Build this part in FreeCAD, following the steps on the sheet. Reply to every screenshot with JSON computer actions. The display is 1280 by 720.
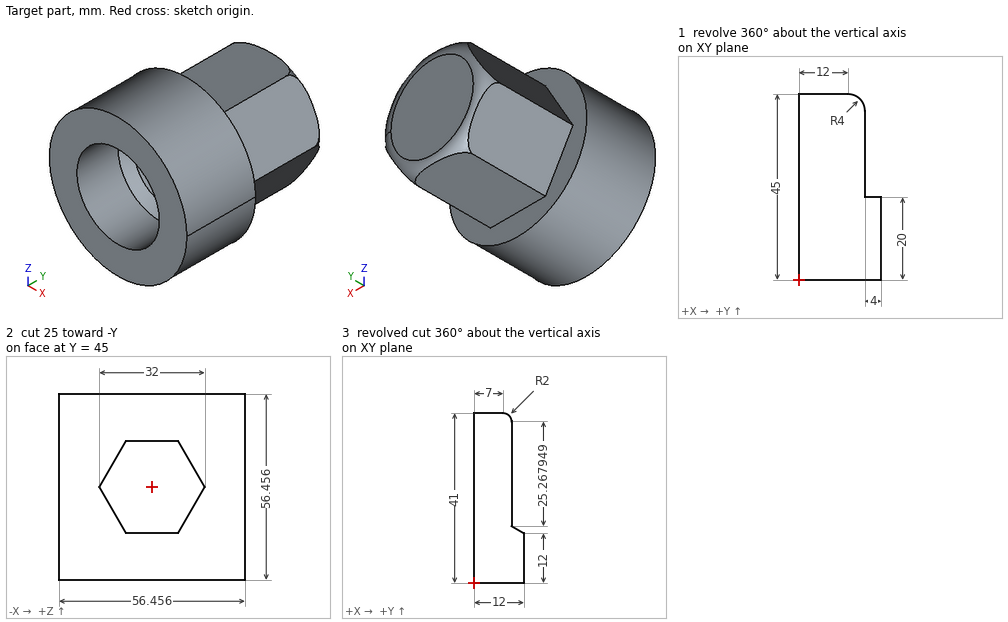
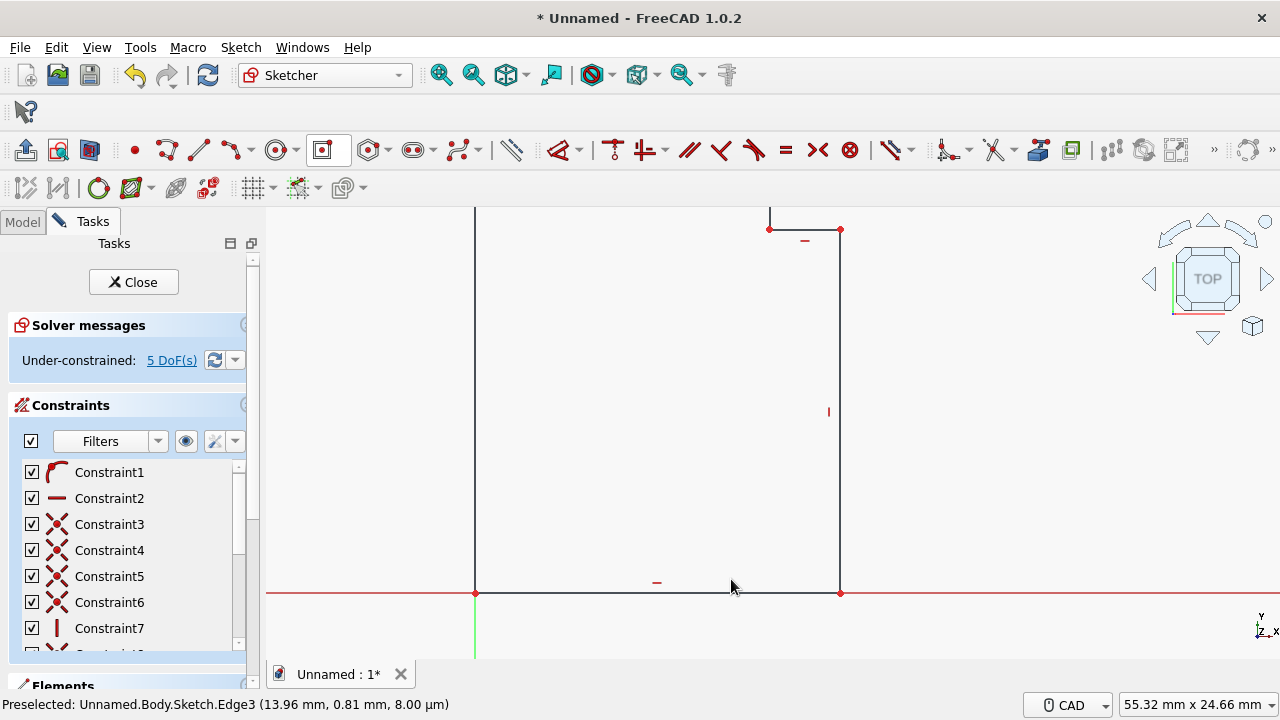
{"action": "key", "text": "d"}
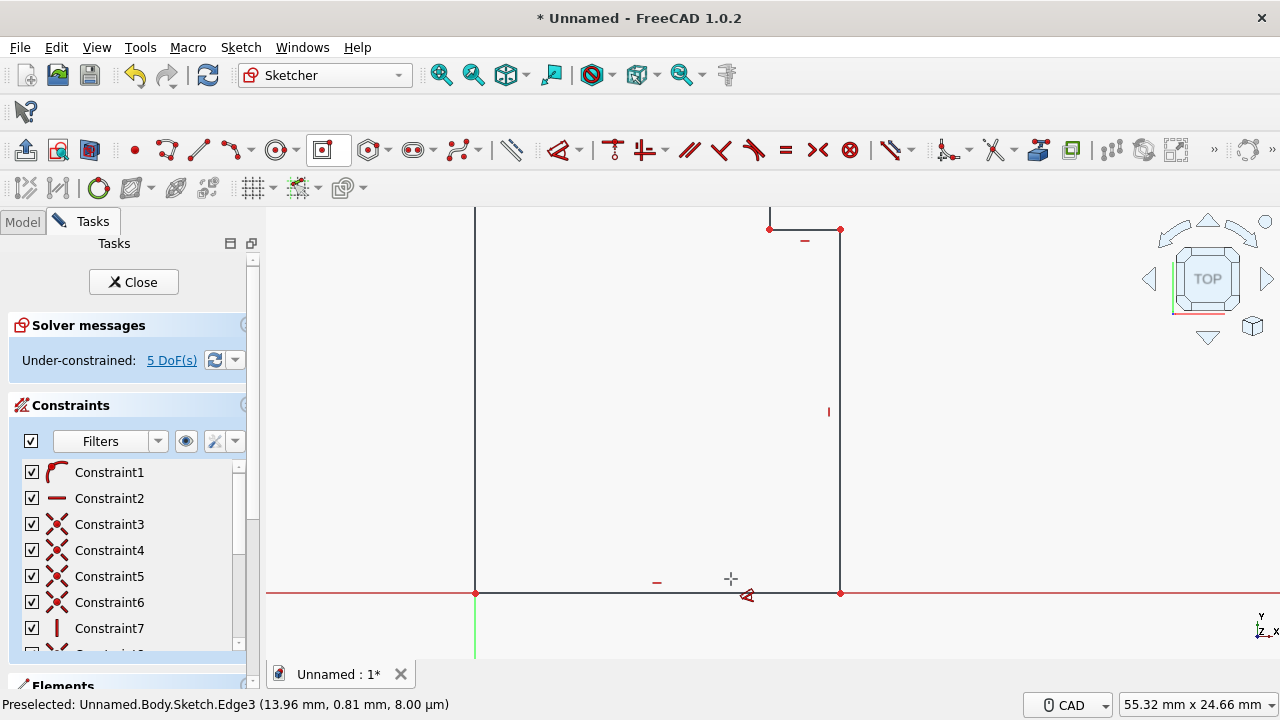
{"action": "scroll", "coordinate": [731, 580], "scroll_direction": "down", "scroll_amount": 5}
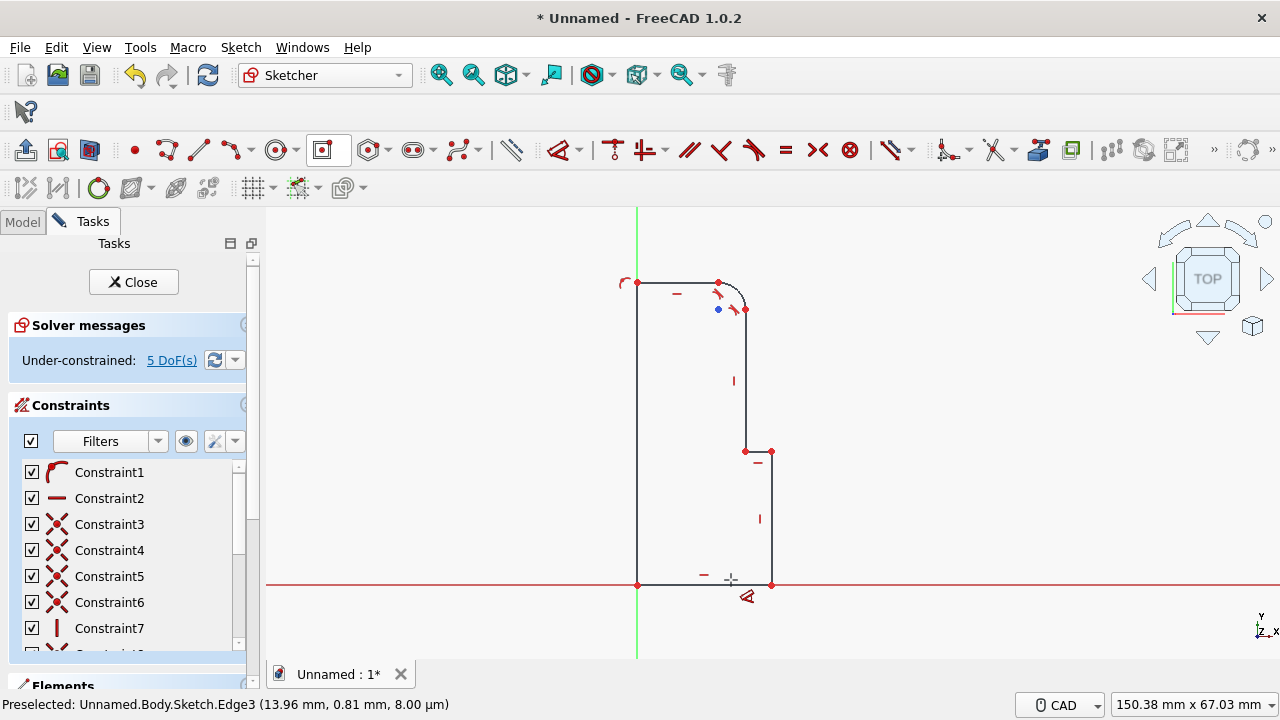
{"action": "scroll", "coordinate": [743, 297], "scroll_direction": "up", "scroll_amount": 2}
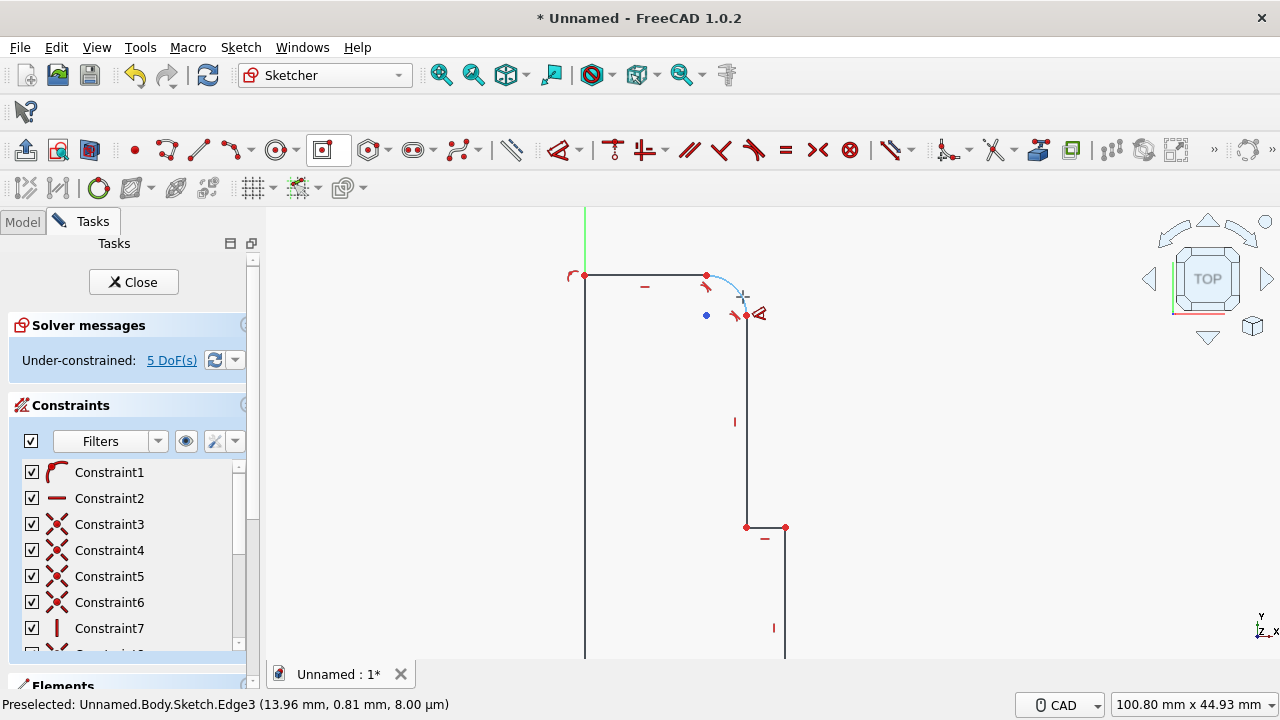
{"action": "left_click", "coordinate": [742, 297]}
{"action": "left_click", "coordinate": [770, 282]}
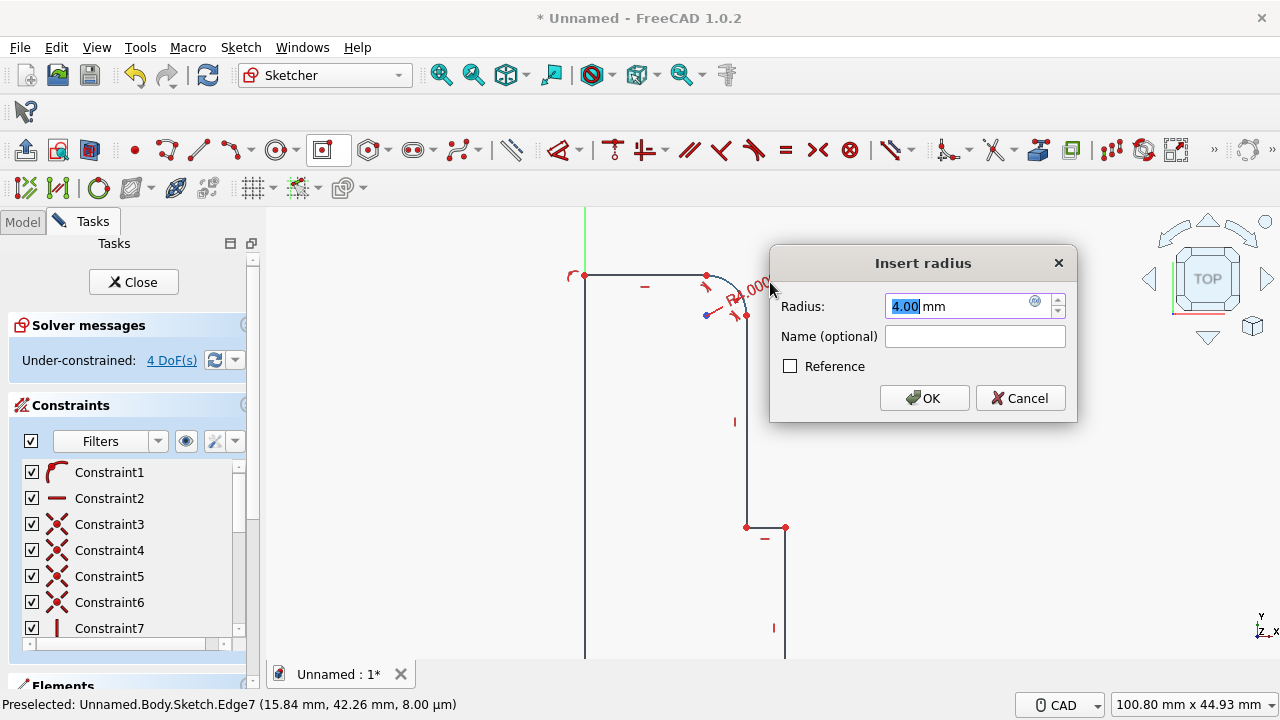
{"action": "type", "text": "4"}
{"action": "key", "text": "Return"}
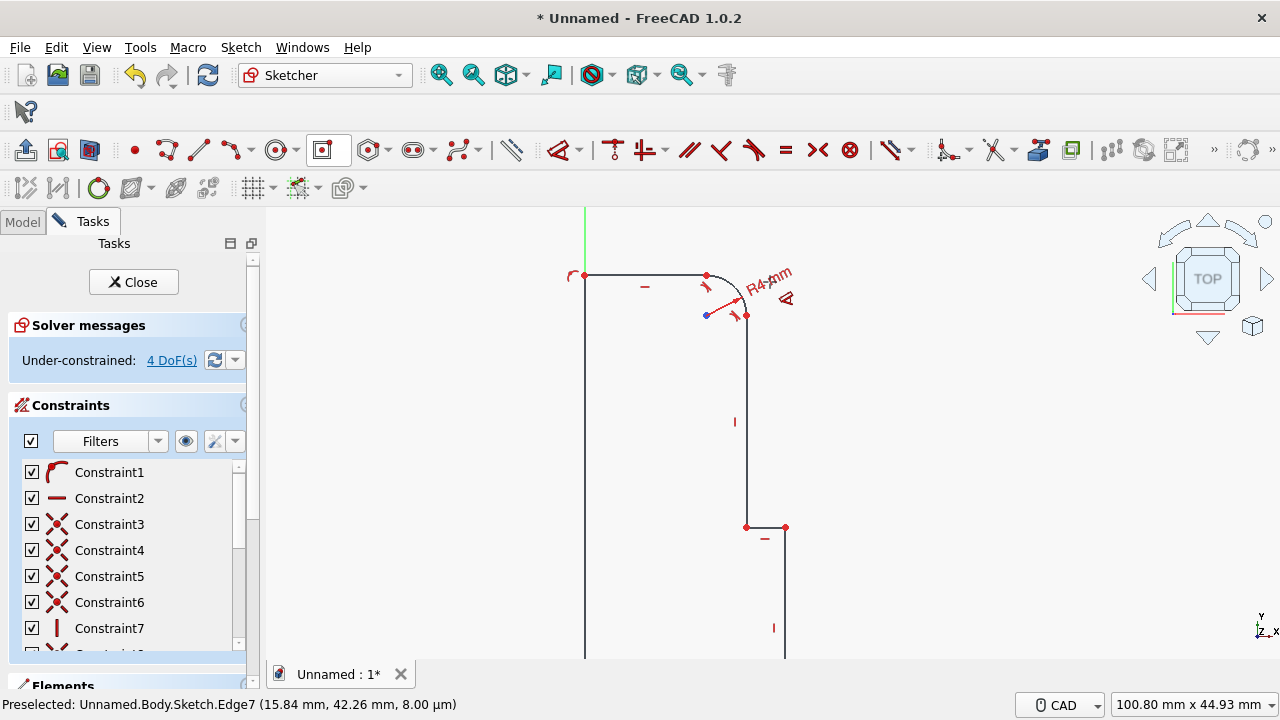
{"action": "left_click", "coordinate": [774, 528]}
{"action": "left_click", "coordinate": [766, 562]}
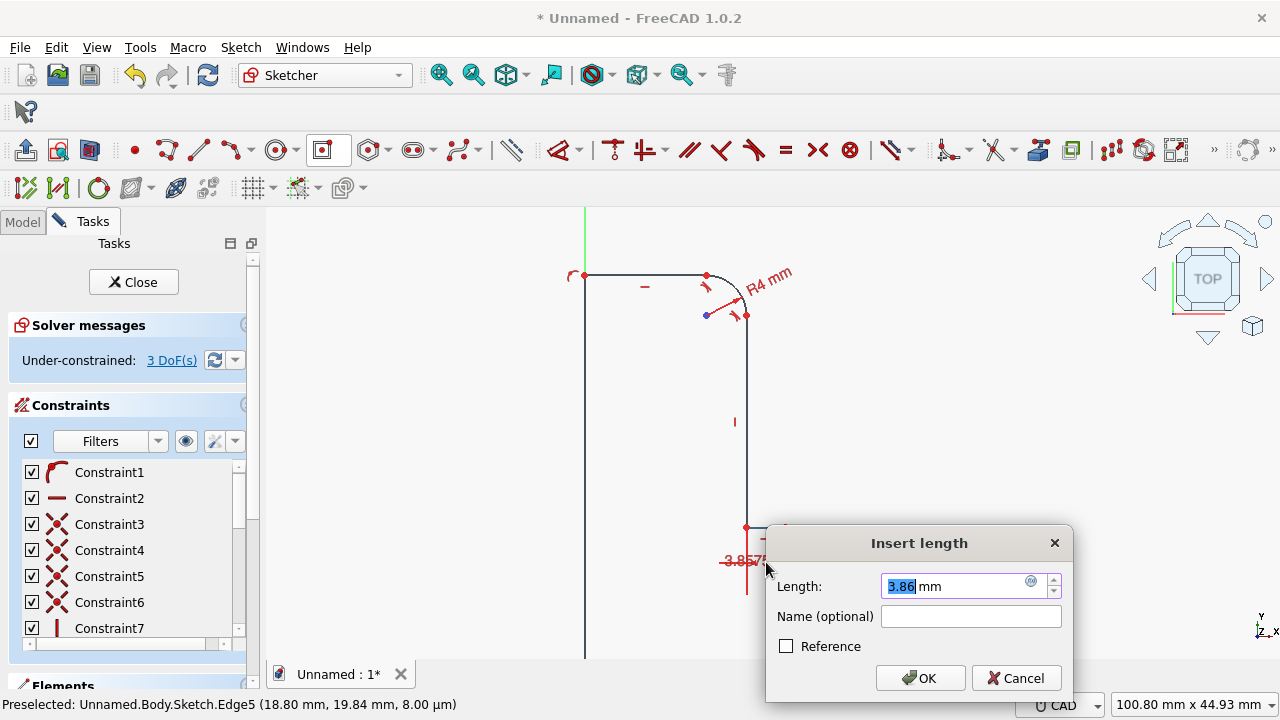
{"action": "type", "text": "4"}
{"action": "key", "text": "Return"}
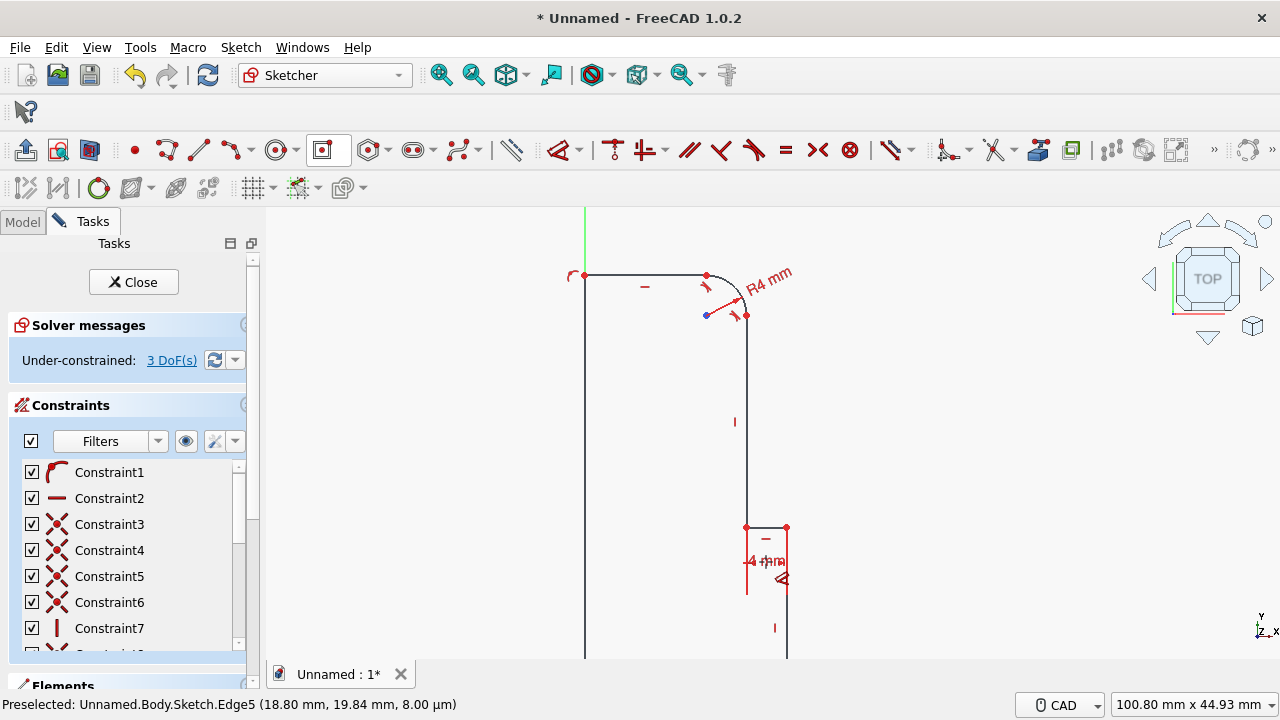
{"action": "left_click", "coordinate": [670, 275]}
{"action": "left_click", "coordinate": [646, 241]}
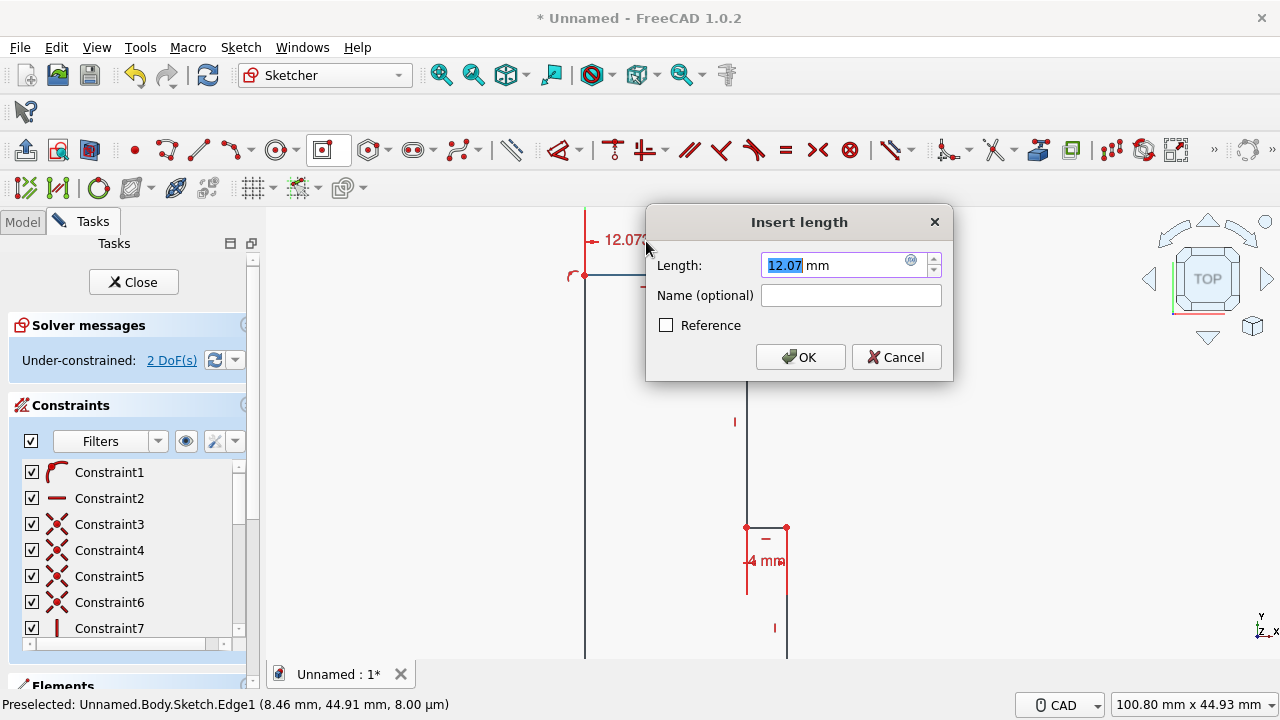
{"action": "type", "text": "12"}
{"action": "key", "text": "Return"}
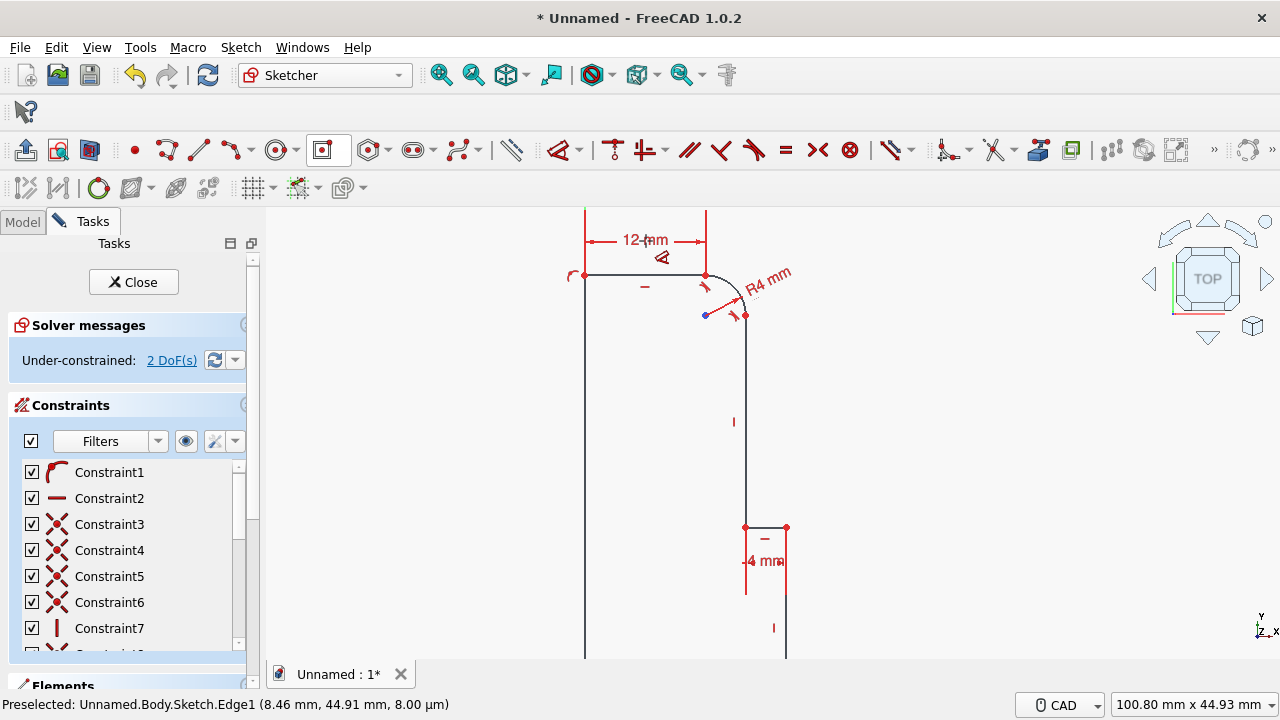
{"action": "left_click", "coordinate": [585, 411]}
{"action": "left_click", "coordinate": [551, 453]}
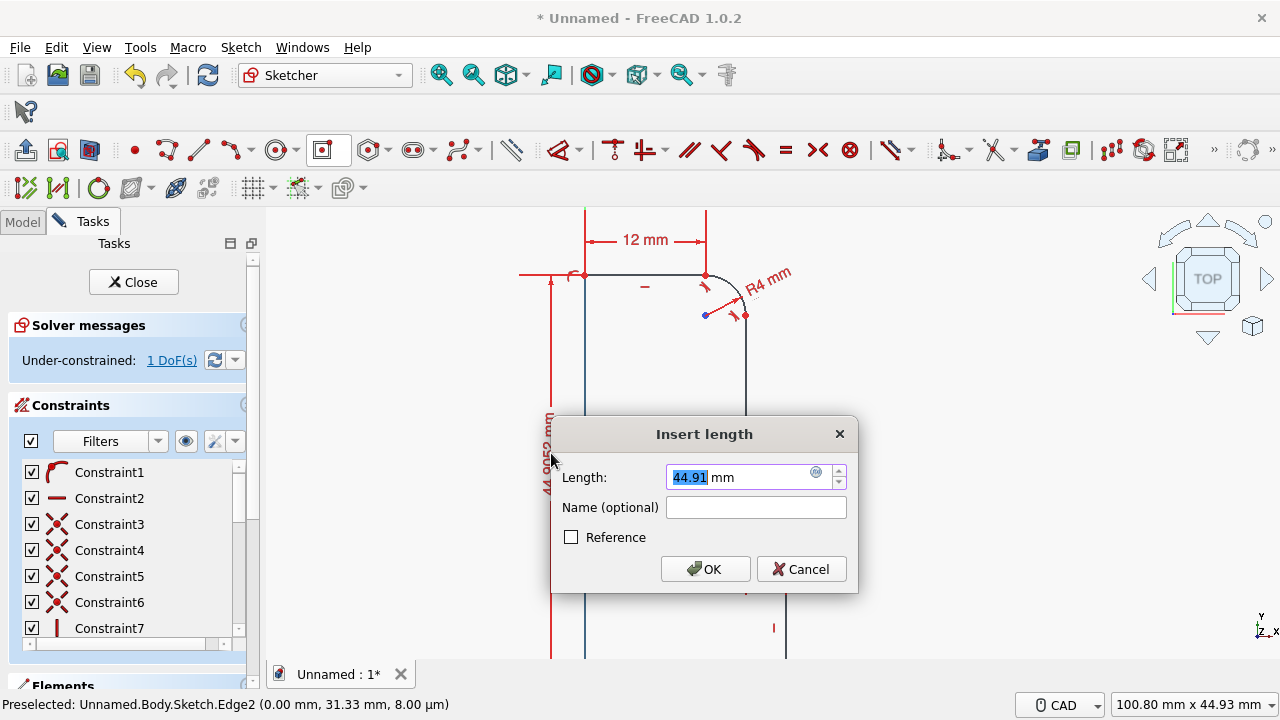
{"action": "type", "text": "45"}
{"action": "key", "text": "Return"}